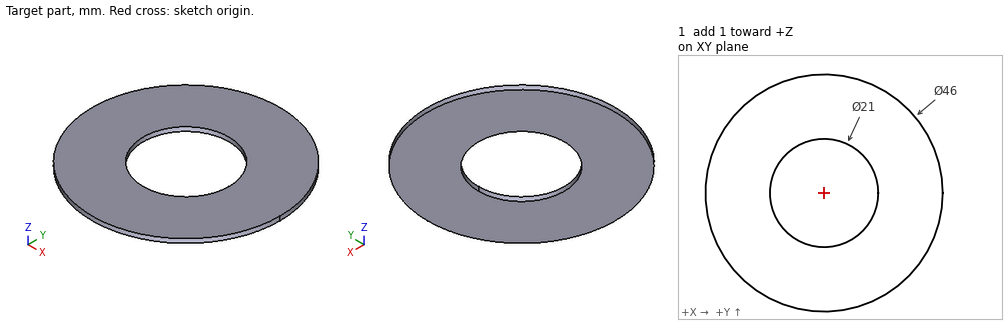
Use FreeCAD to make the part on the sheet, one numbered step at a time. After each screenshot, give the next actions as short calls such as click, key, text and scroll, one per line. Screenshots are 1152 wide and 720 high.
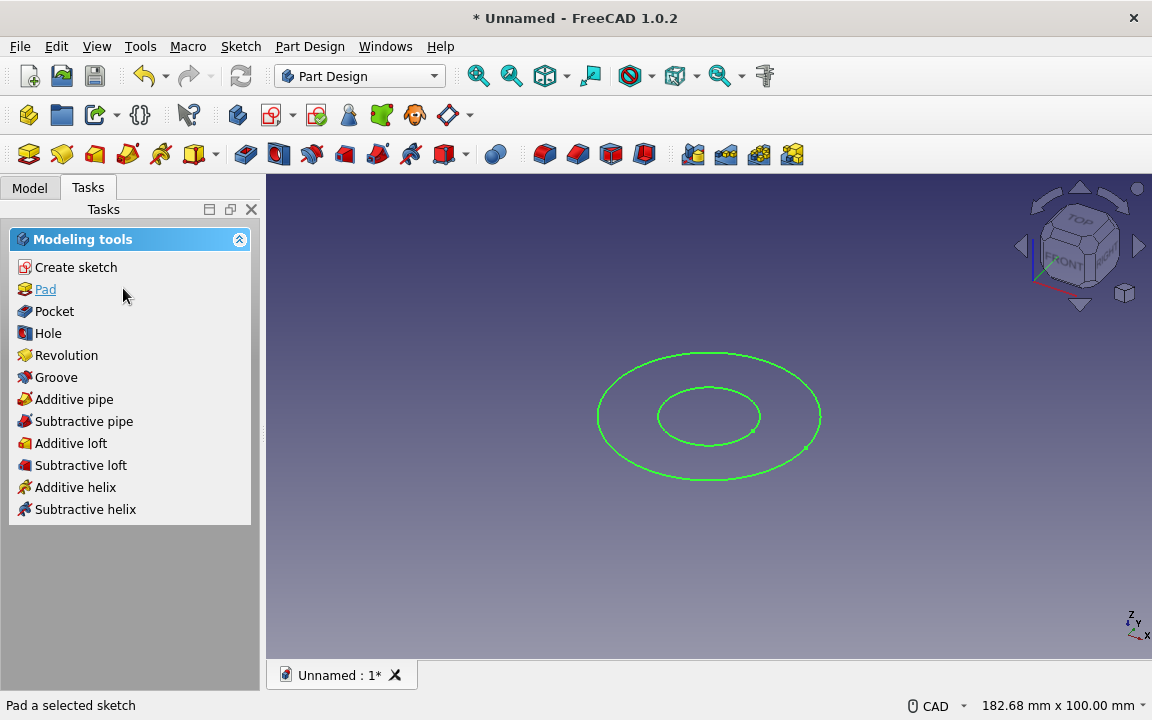
click(29, 154)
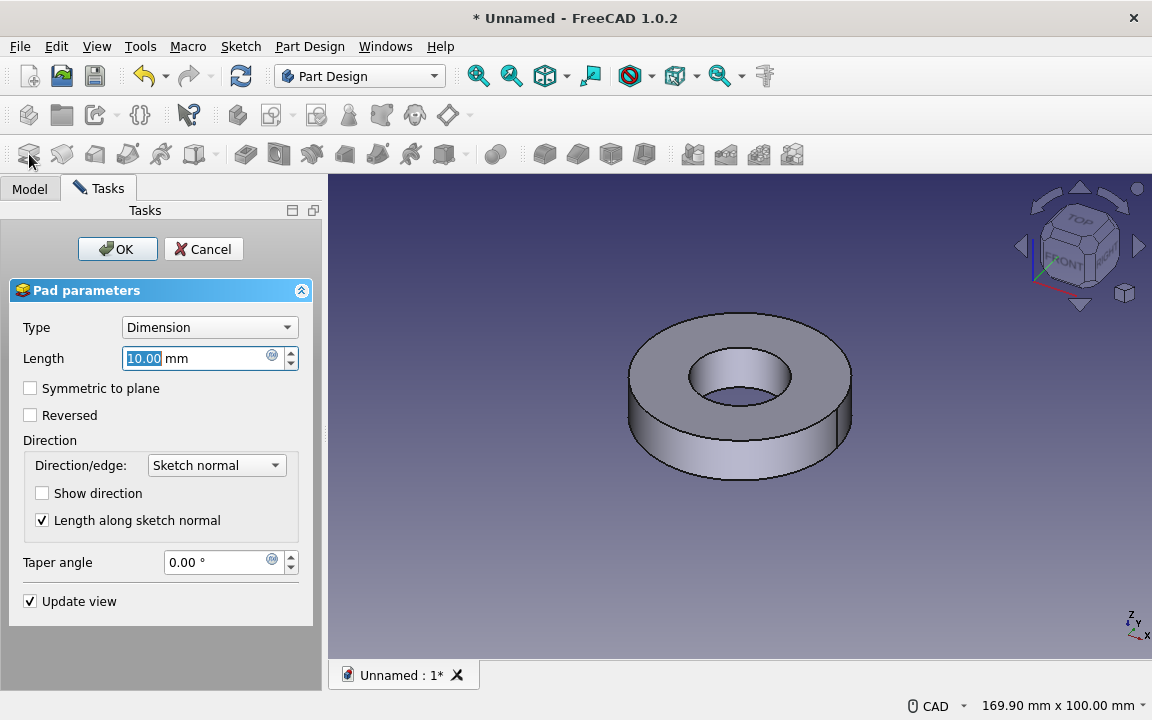
text(1)
key(Tab)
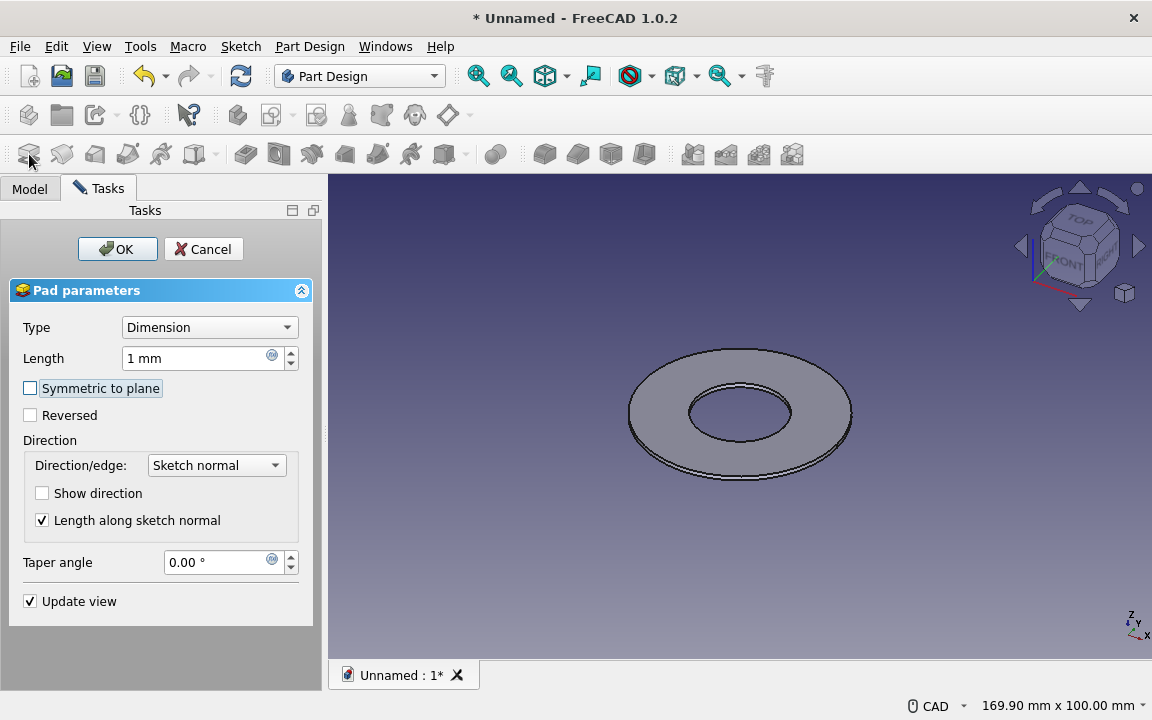
click(118, 249)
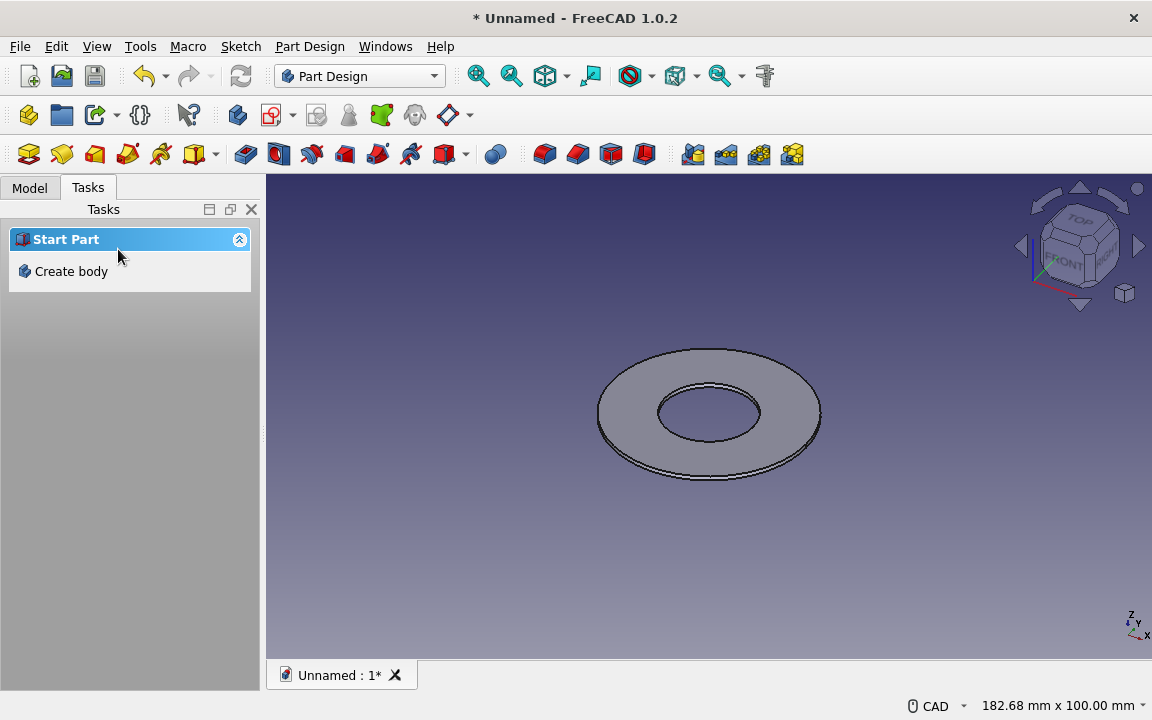
key(0)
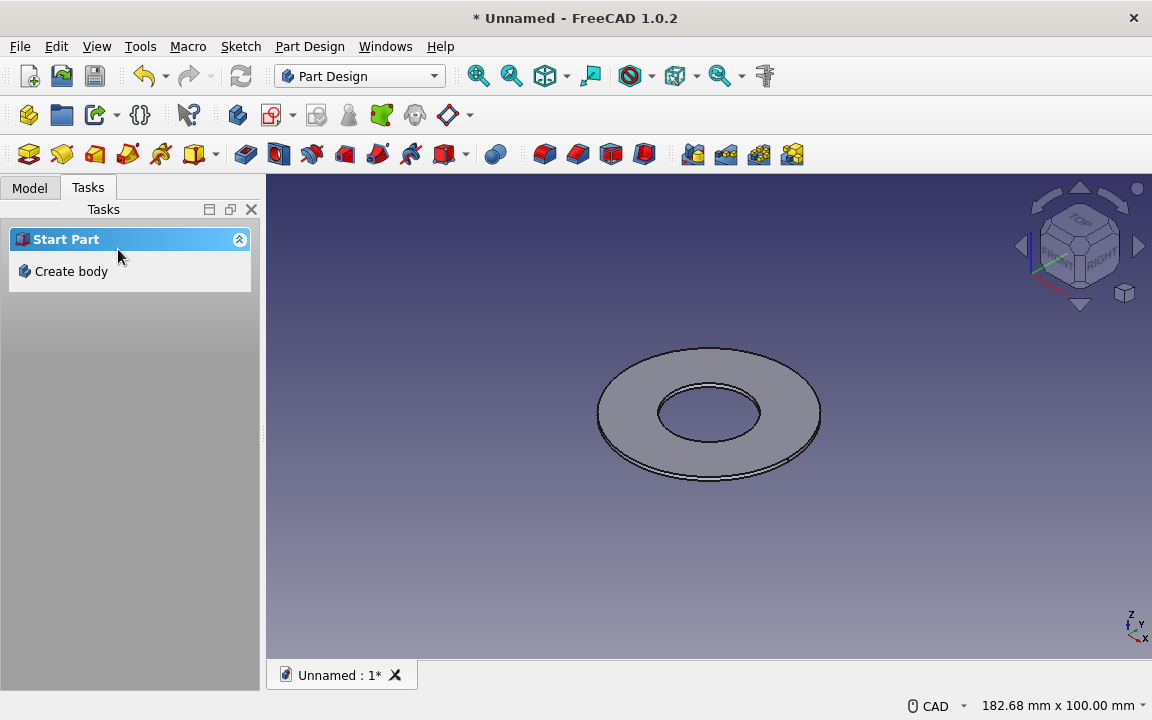
key(v)
key(f)